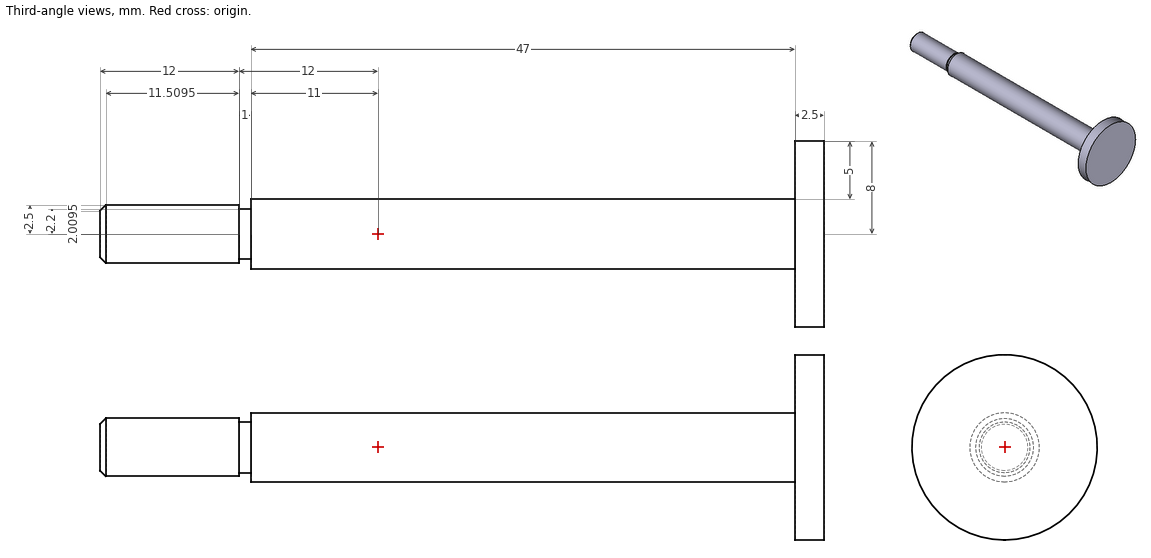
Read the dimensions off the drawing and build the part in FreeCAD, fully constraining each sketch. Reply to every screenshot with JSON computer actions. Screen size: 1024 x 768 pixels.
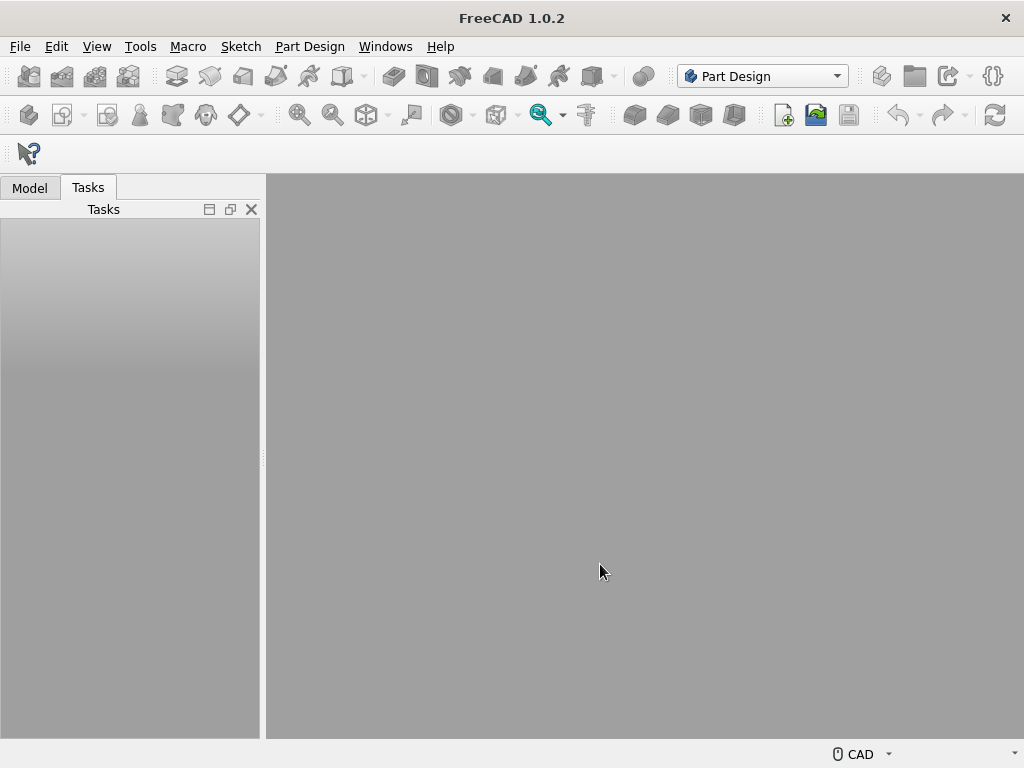
{"action": "left_click", "coordinate": [783, 116]}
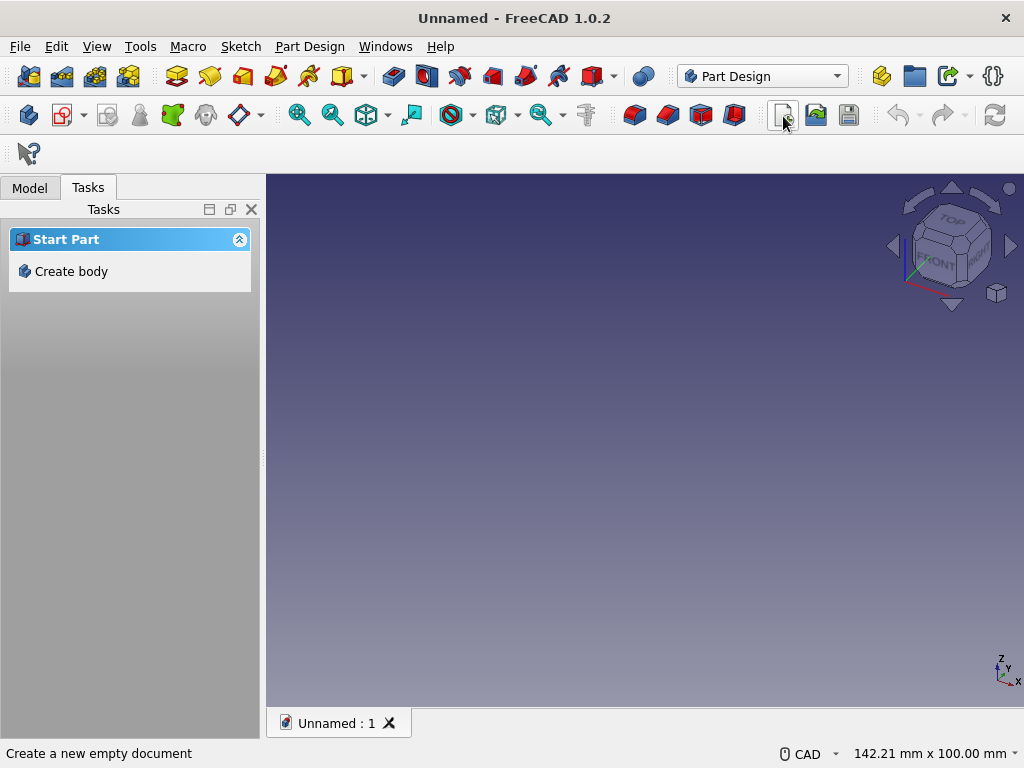
{"action": "left_click", "coordinate": [62, 116]}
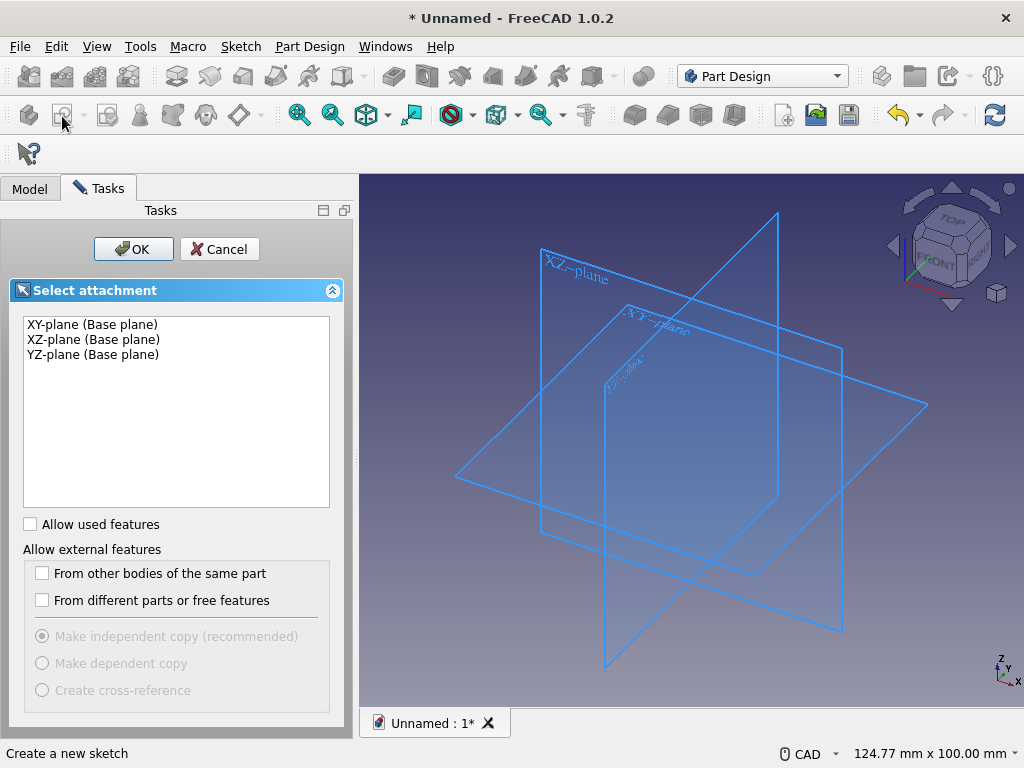
{"action": "left_click", "coordinate": [84, 324]}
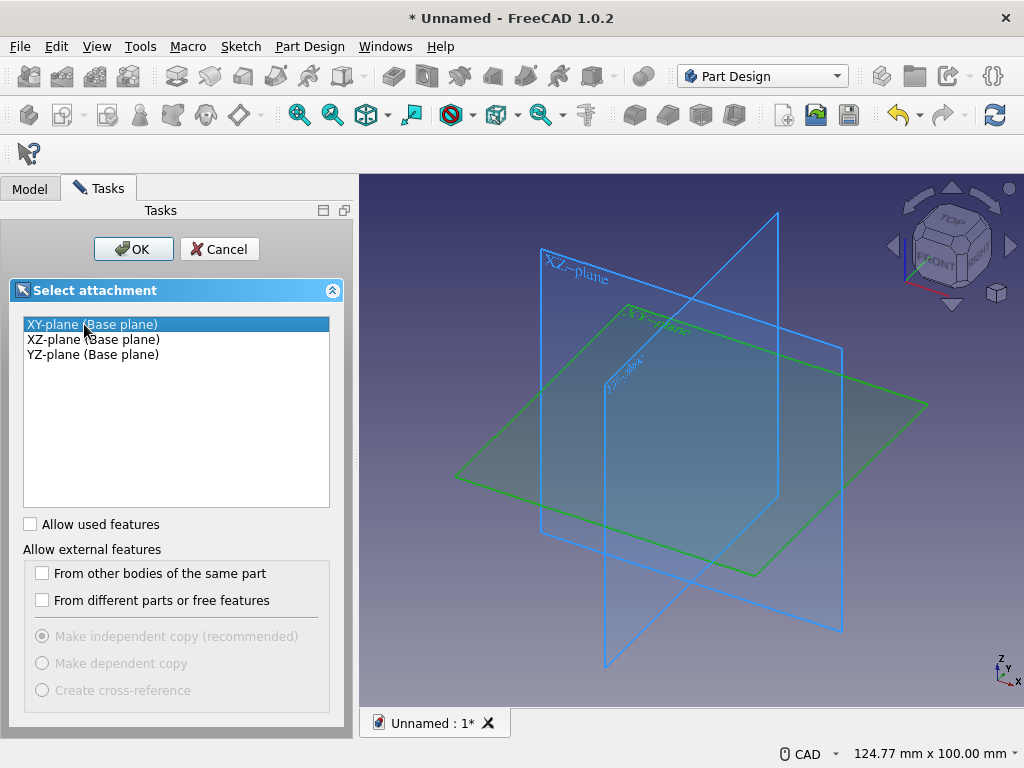
{"action": "left_click", "coordinate": [134, 249]}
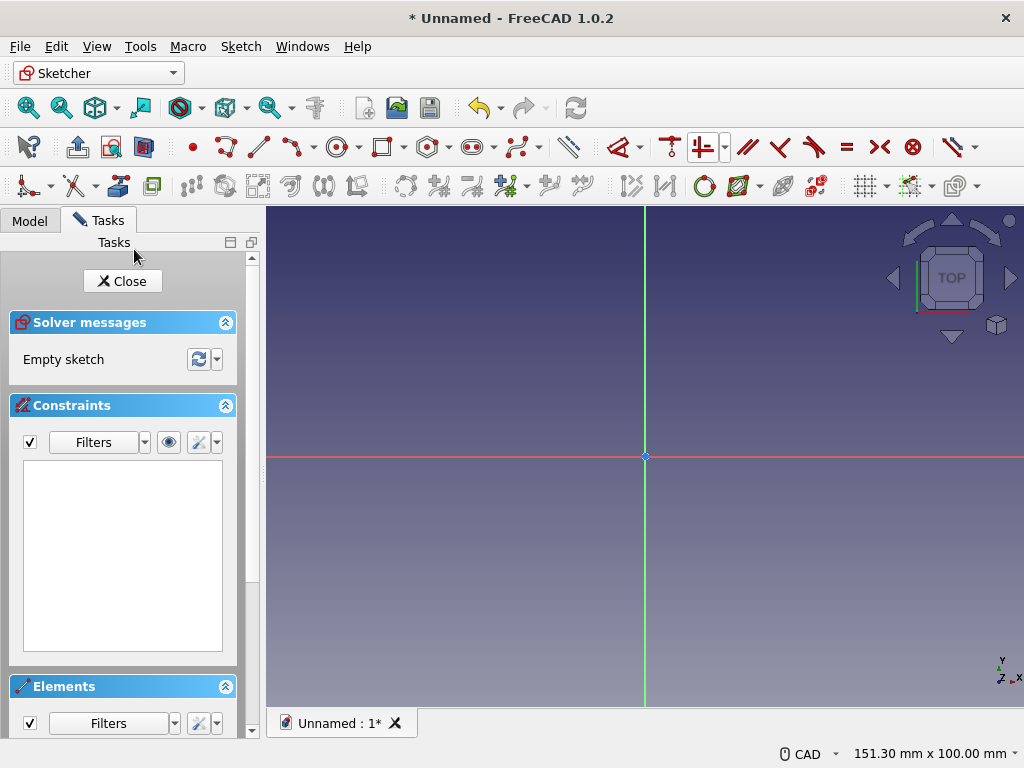
{"action": "scroll", "coordinate": [859, 396], "scroll_direction": "up", "scroll_amount": 2}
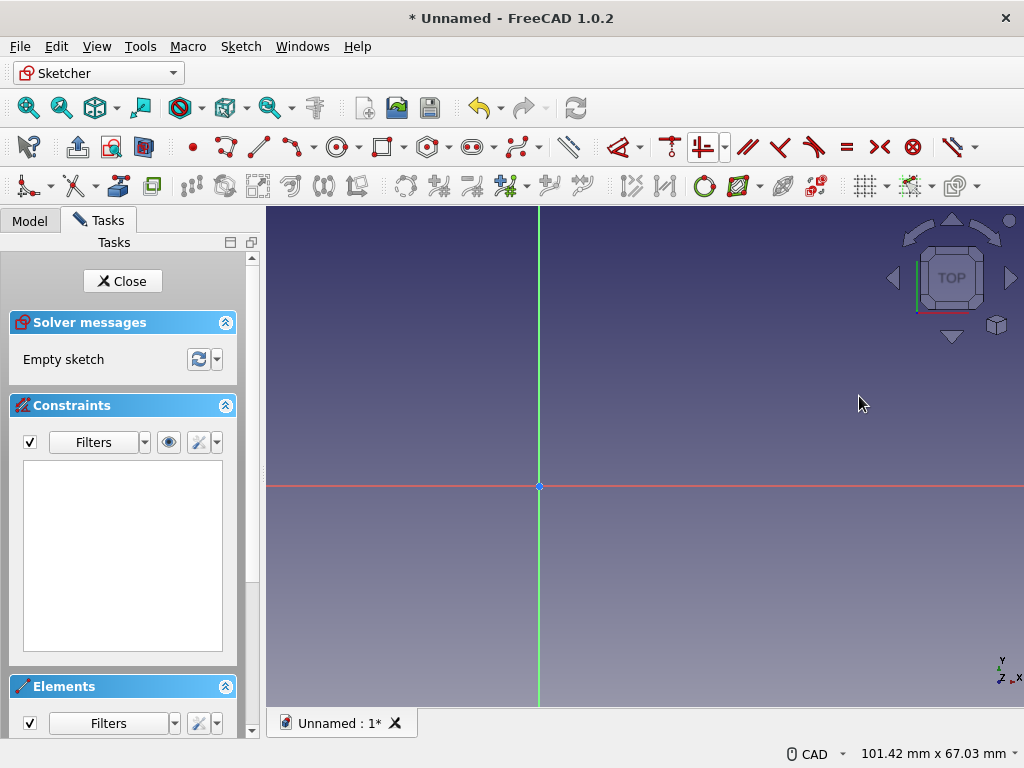
{"action": "left_click", "coordinate": [226, 148]}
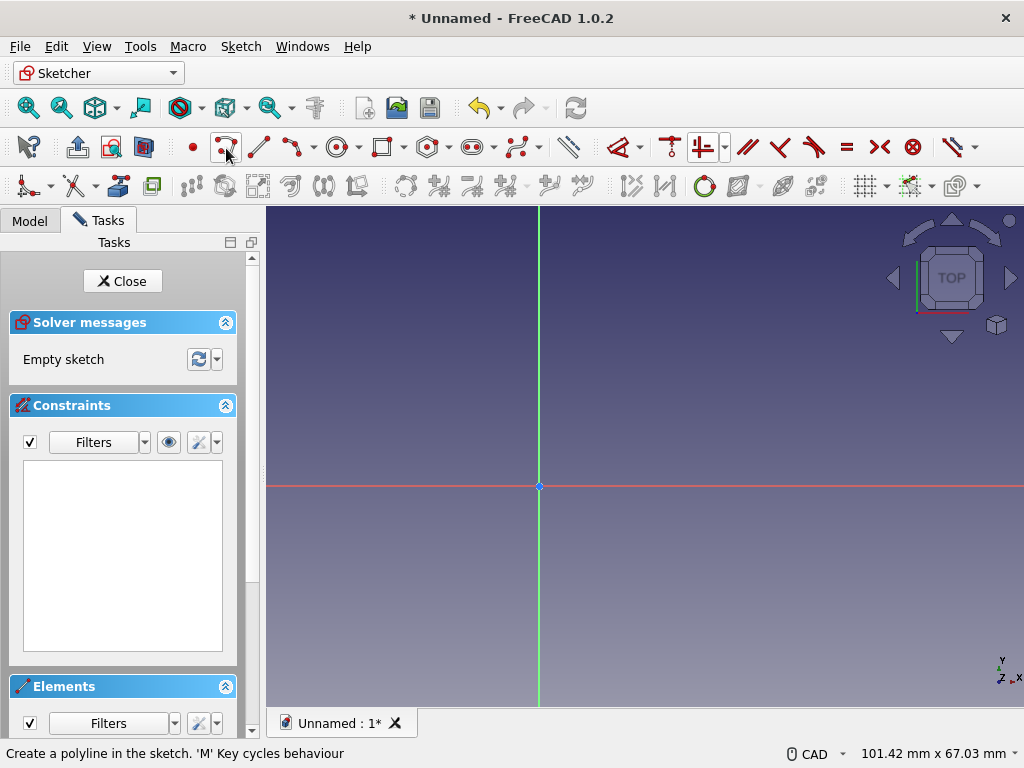
{"action": "left_click", "coordinate": [457, 486]}
{"action": "left_click", "coordinate": [827, 477]}
{"action": "left_click", "coordinate": [827, 426]}
{"action": "left_click", "coordinate": [808, 426]}
{"action": "left_click", "coordinate": [808, 464]}
{"action": "left_click", "coordinate": [457, 464]}
{"action": "left_click", "coordinate": [457, 486]}
{"action": "key", "text": "Escape"}
{"action": "key", "text": "Escape"}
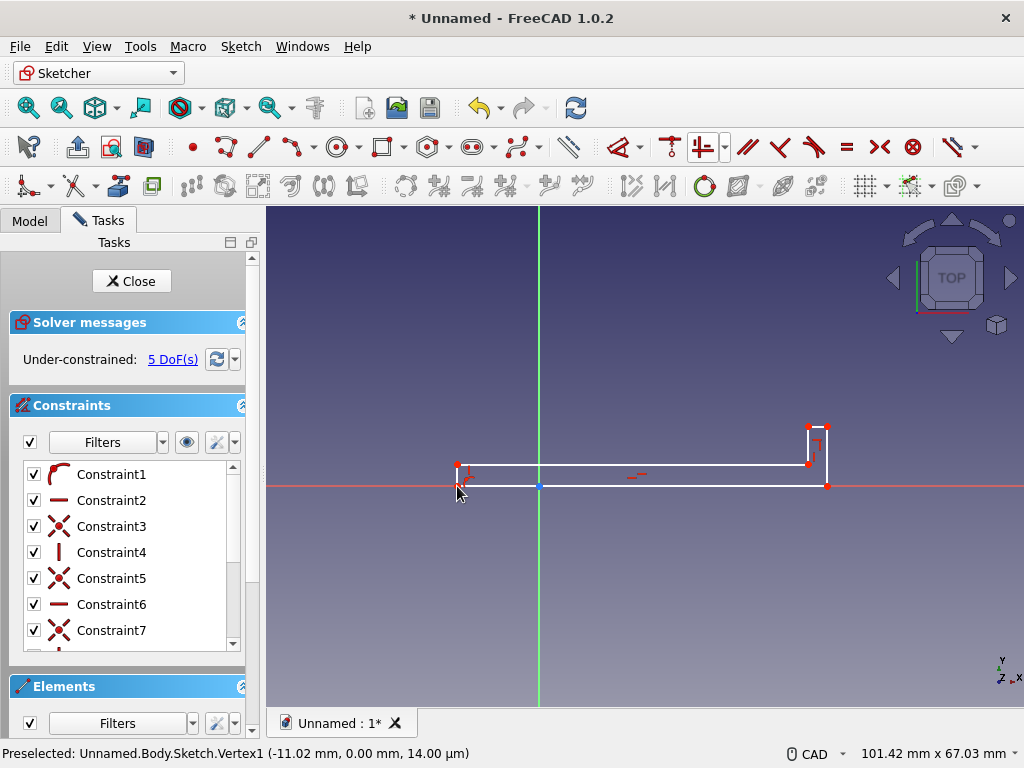
{"action": "left_click", "coordinate": [618, 148]}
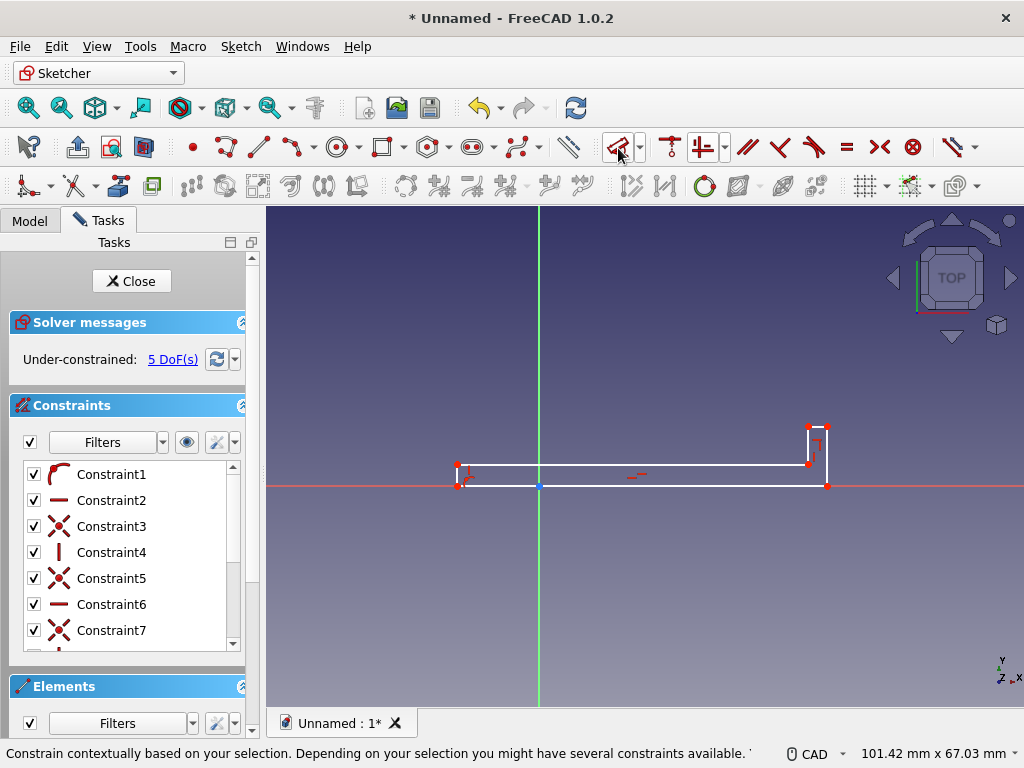
{"action": "left_click", "coordinate": [827, 468]}
{"action": "left_click", "coordinate": [793, 443]}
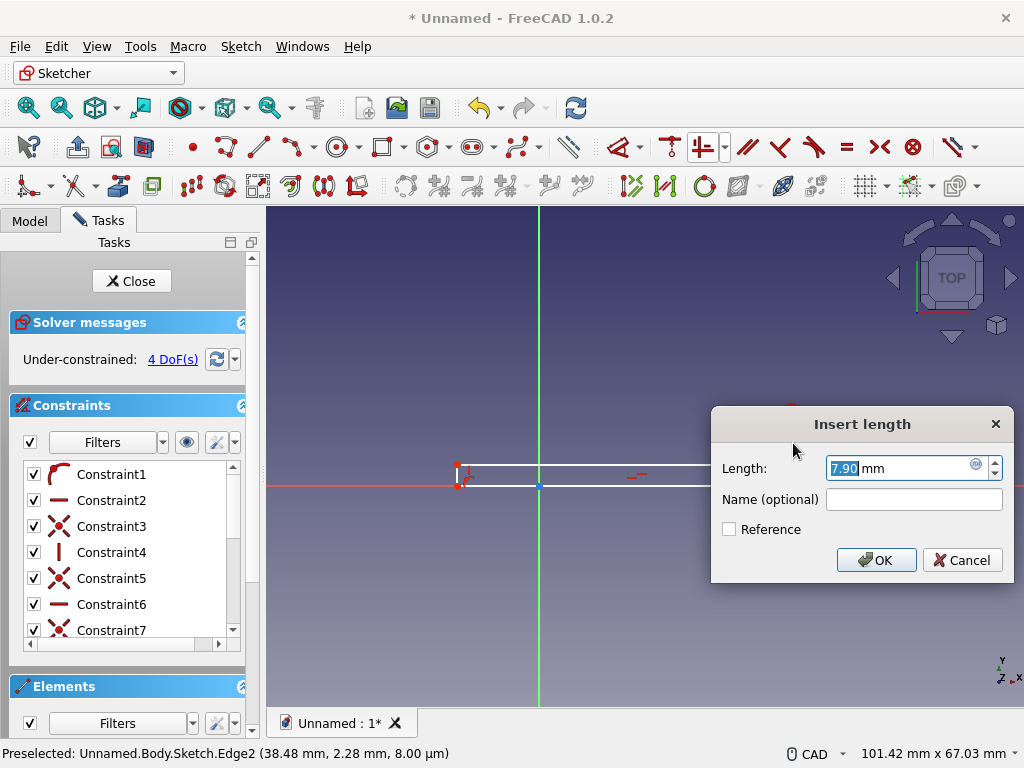
{"action": "type", "text": "8"}
{"action": "key", "text": "Return"}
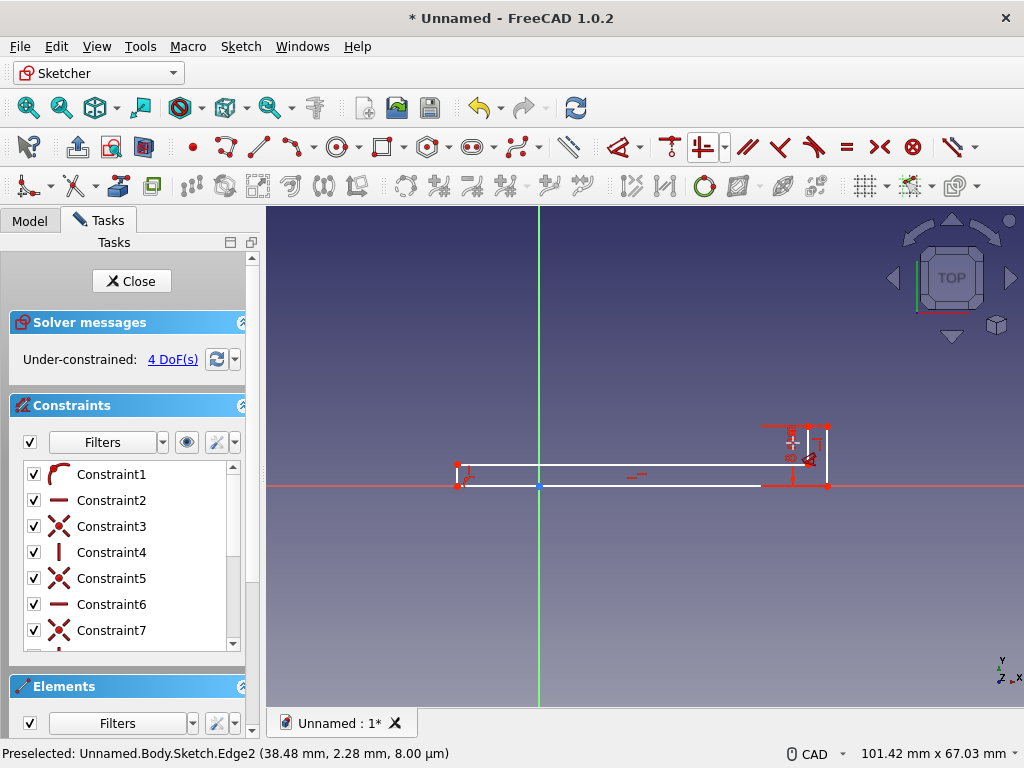
{"action": "left_click", "coordinate": [808, 438]}
{"action": "left_click", "coordinate": [702, 446]}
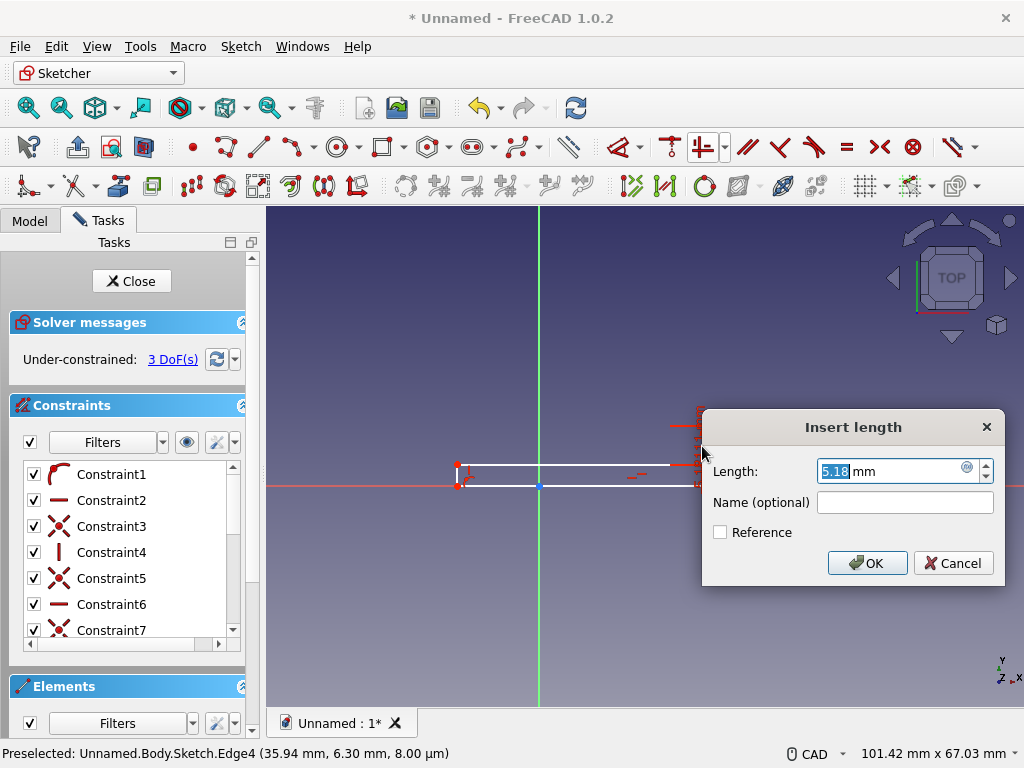
{"action": "type", "text": "5"}
{"action": "key", "text": "Return"}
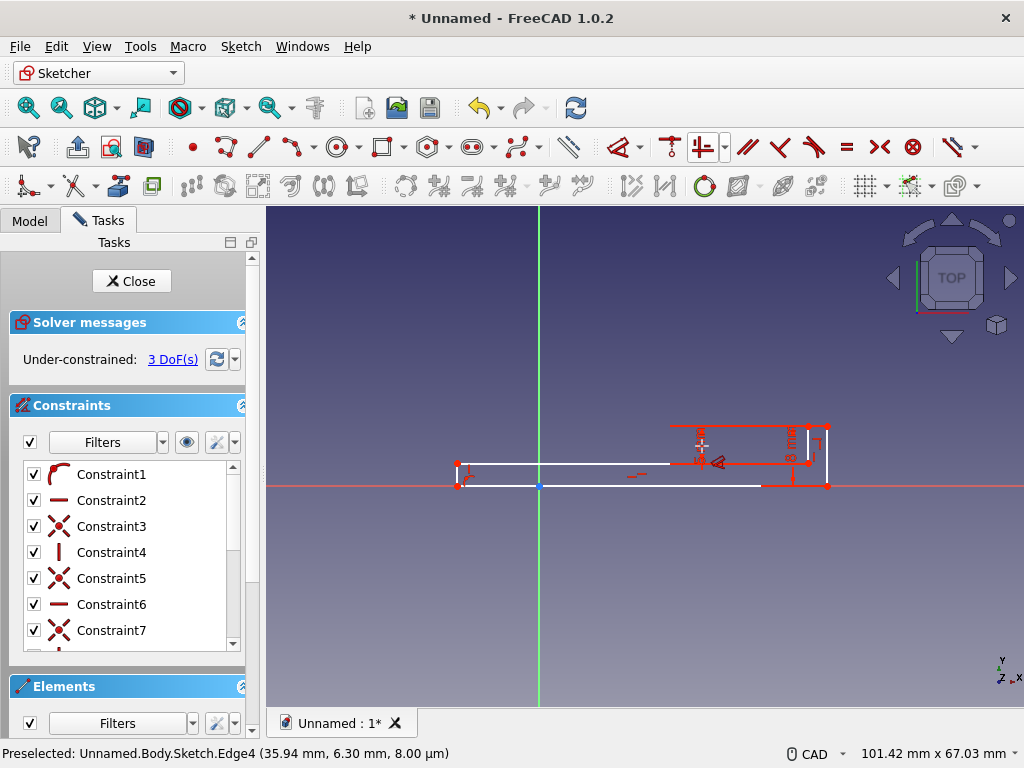
{"action": "left_click", "coordinate": [703, 464]}
{"action": "left_click", "coordinate": [510, 430]}